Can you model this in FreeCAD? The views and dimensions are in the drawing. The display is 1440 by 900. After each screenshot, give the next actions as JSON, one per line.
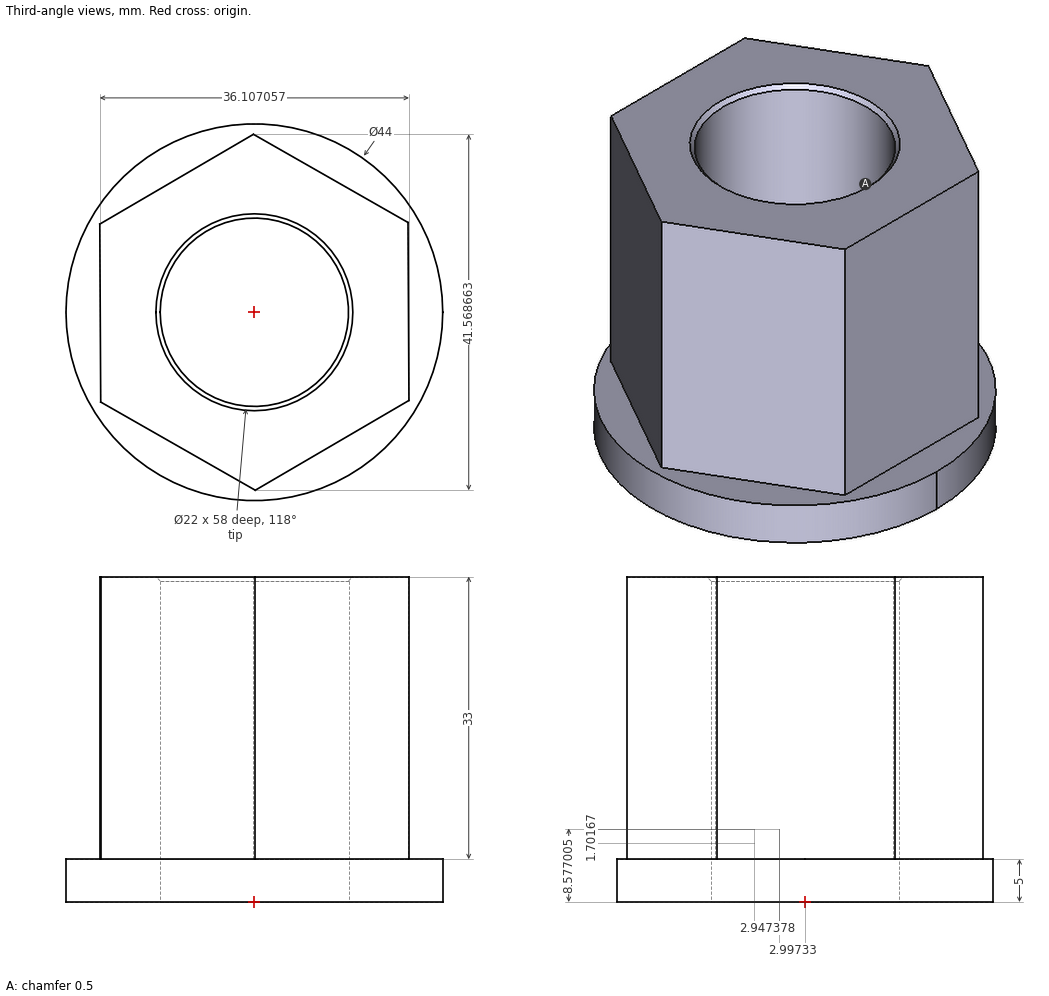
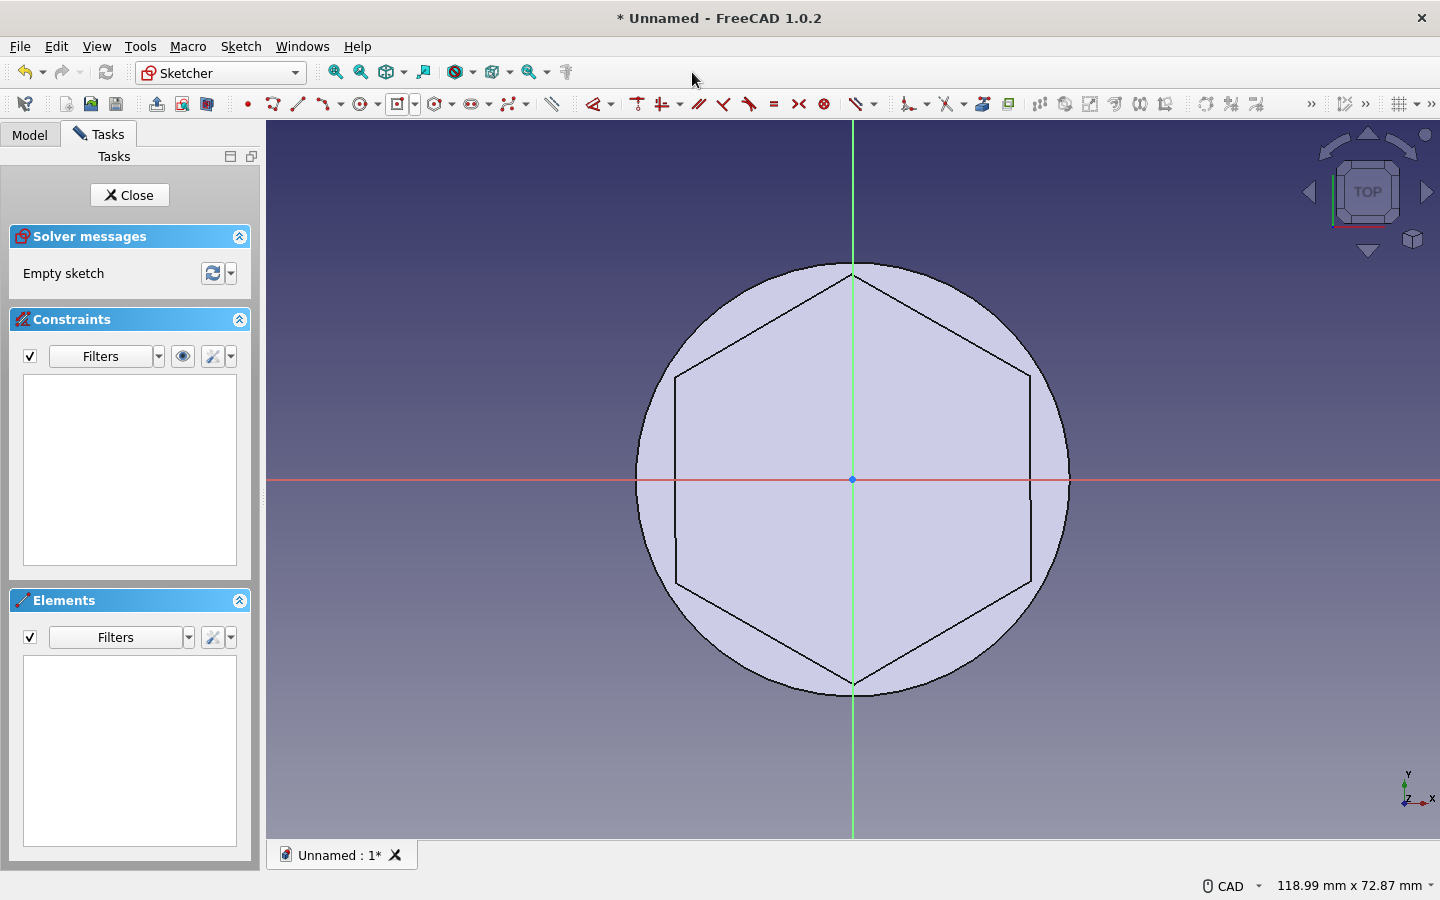
{"action": "scroll", "coordinate": [909, 480], "scroll_direction": "up", "scroll_amount": 4}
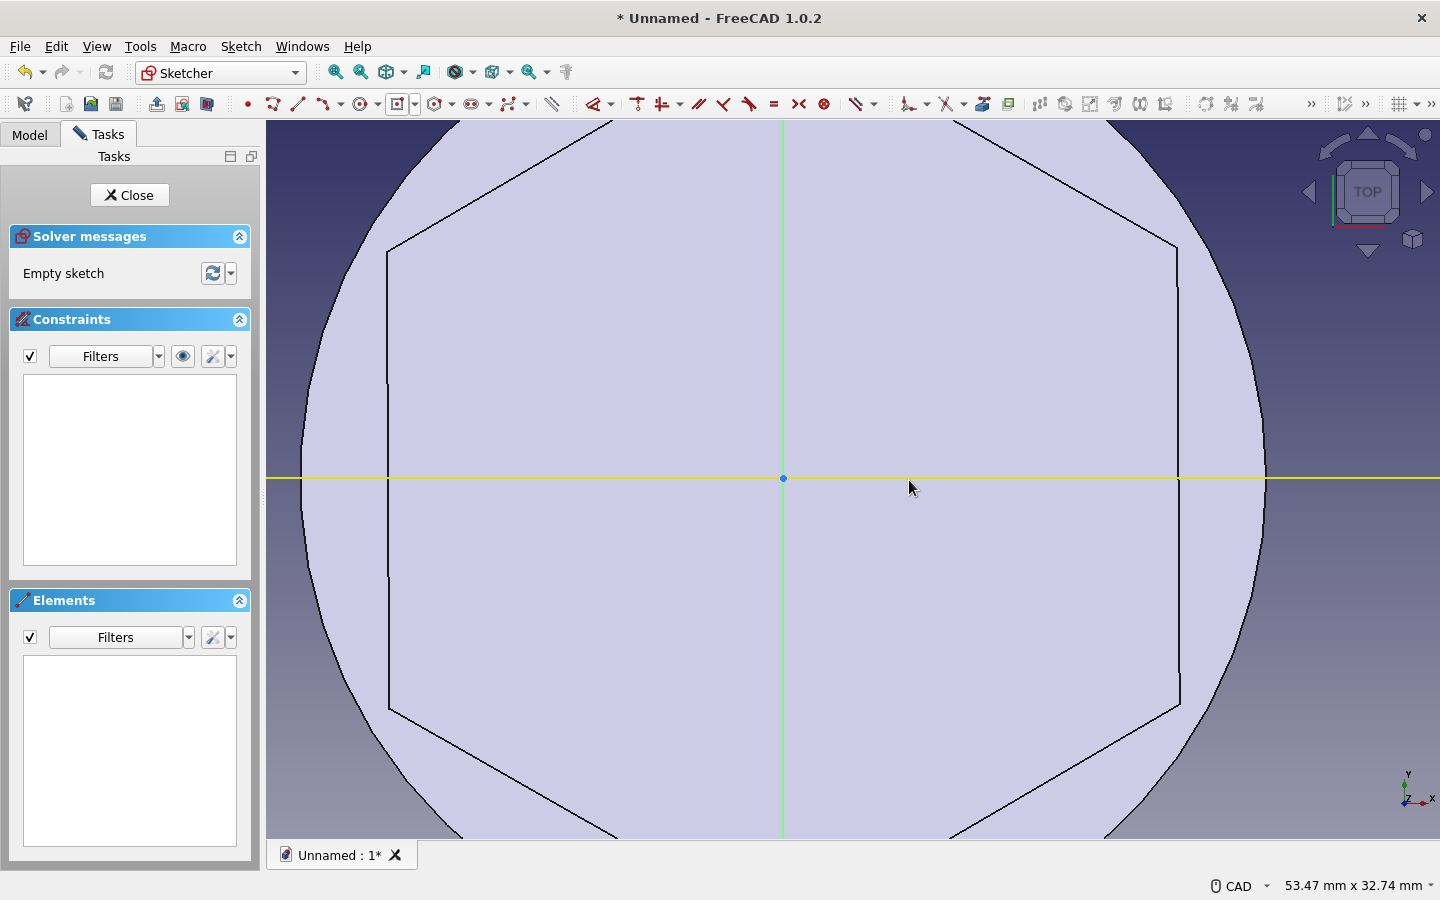
{"action": "left_click", "coordinate": [360, 104]}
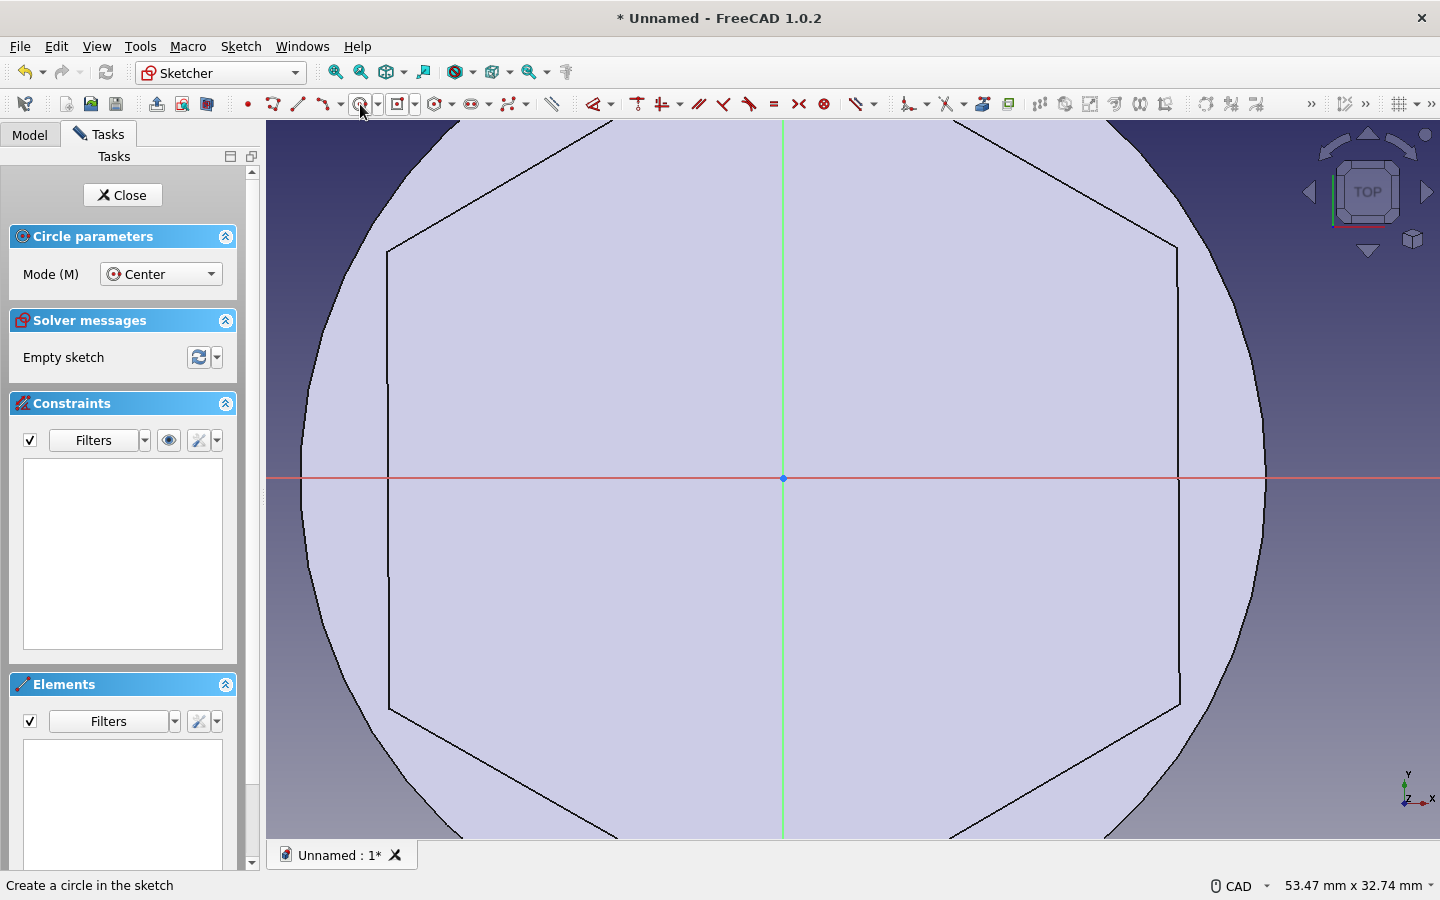
{"action": "left_click", "coordinate": [783, 478]}
{"action": "mouse_move", "coordinate": [954, 307]}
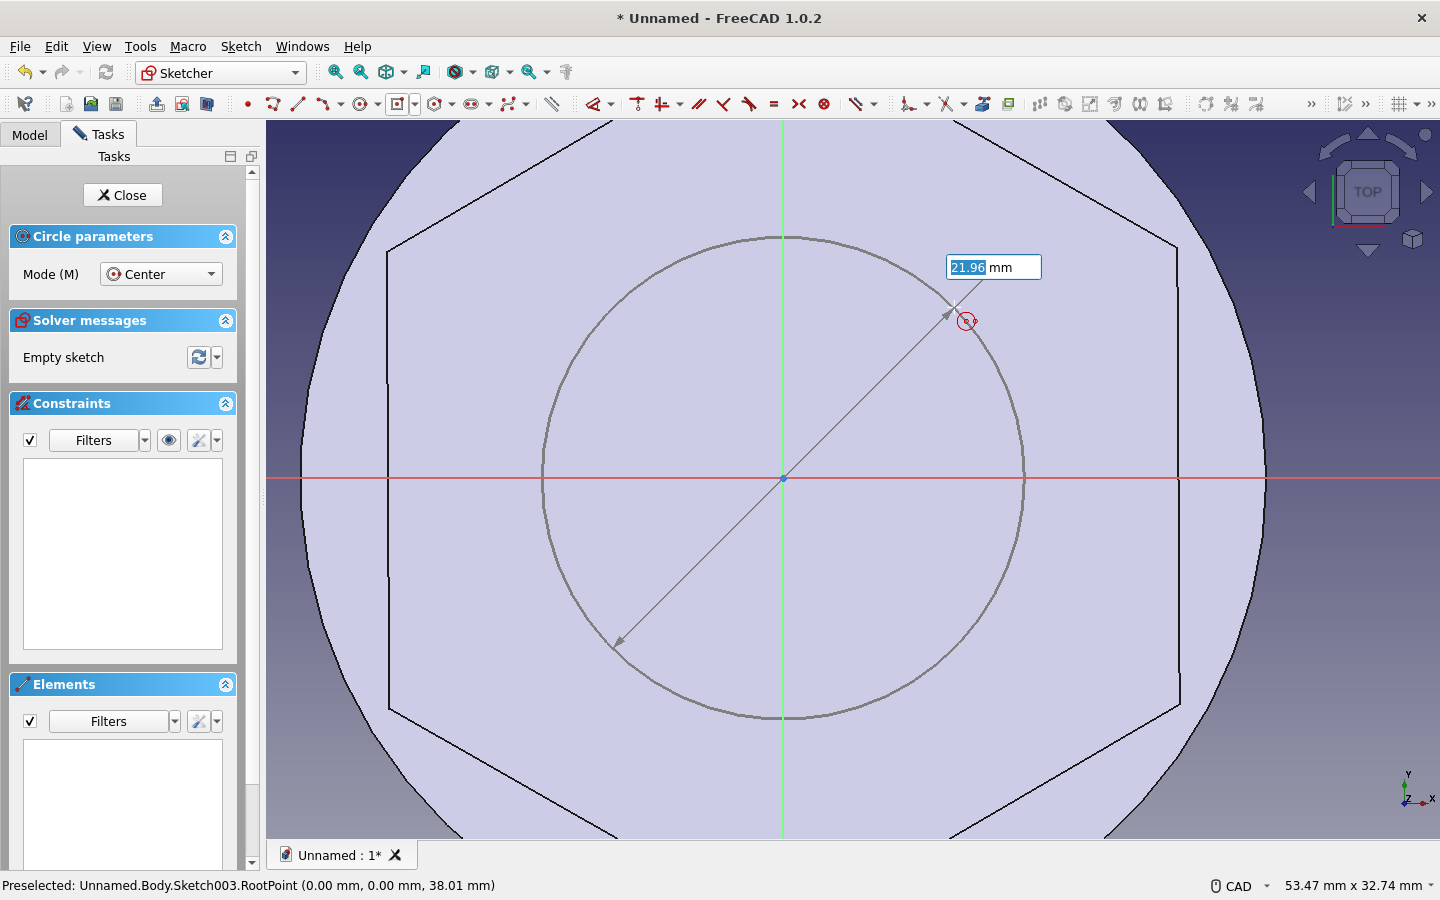
{"action": "type", "text": "22"}
{"action": "key", "text": "Return"}
{"action": "key", "text": "Escape"}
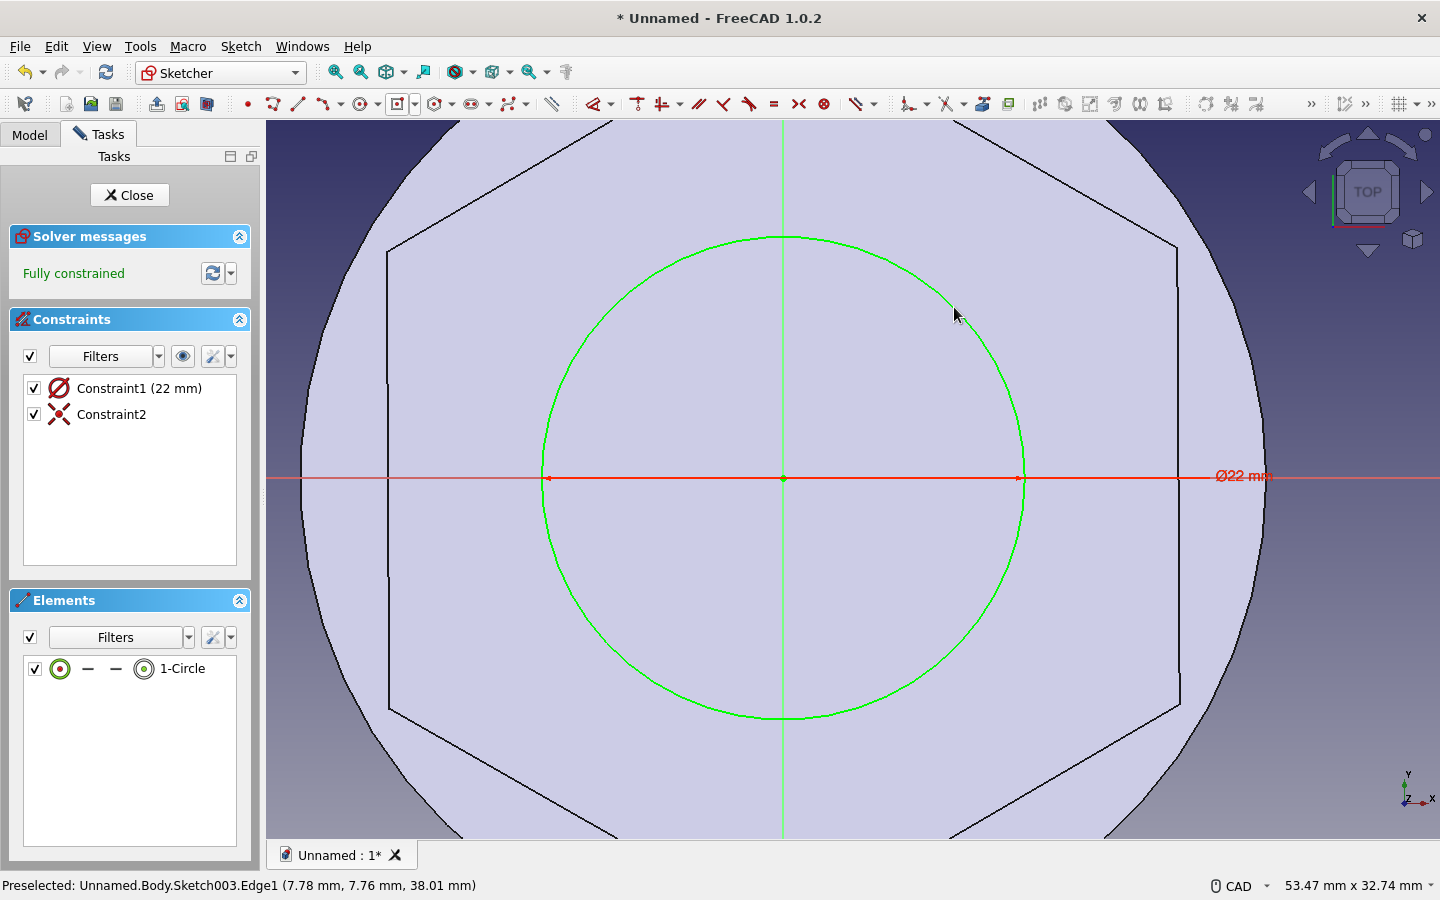
{"action": "left_click", "coordinate": [130, 195]}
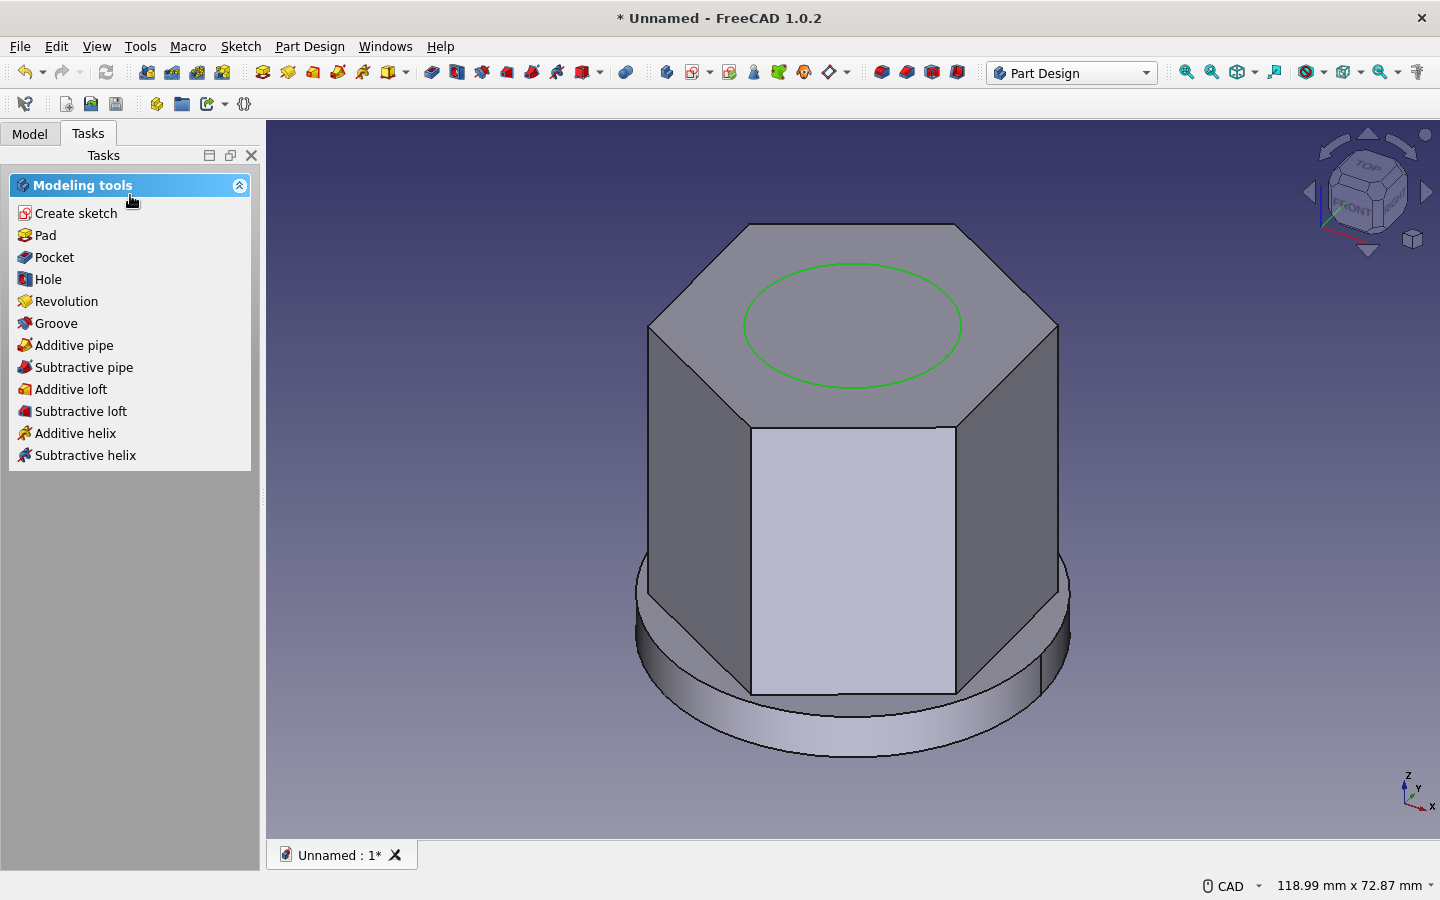
{"action": "left_click", "coordinate": [457, 72]}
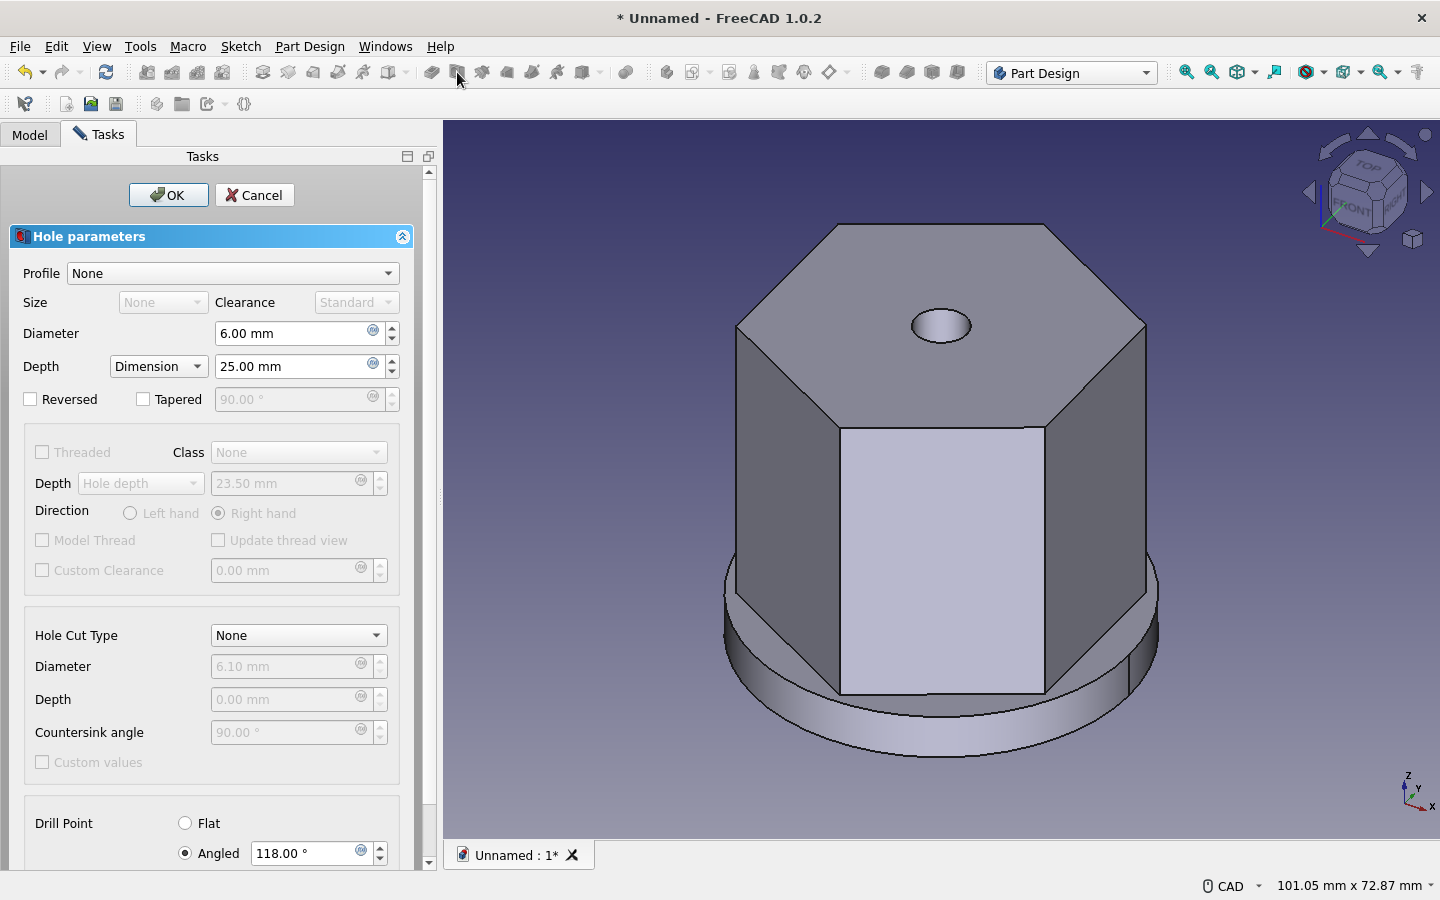
{"action": "triple_click", "coordinate": [300, 334]}